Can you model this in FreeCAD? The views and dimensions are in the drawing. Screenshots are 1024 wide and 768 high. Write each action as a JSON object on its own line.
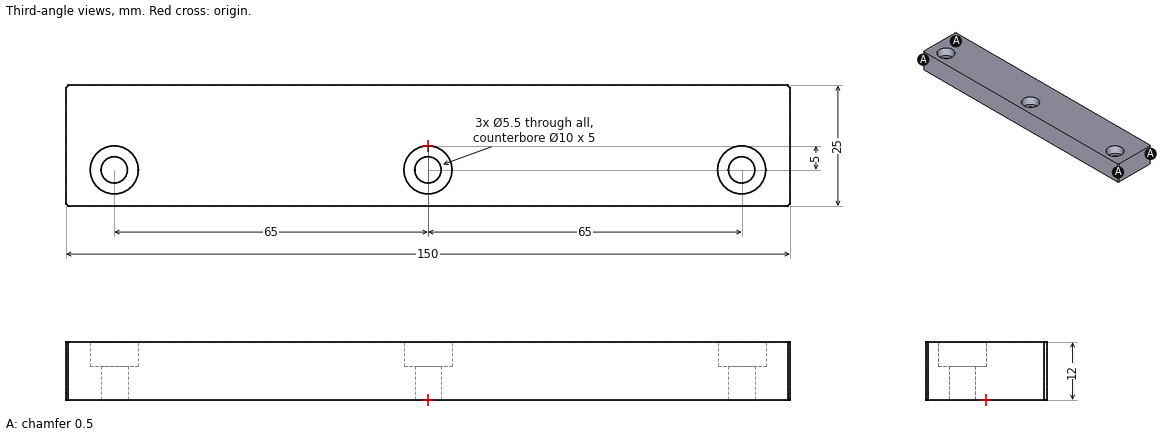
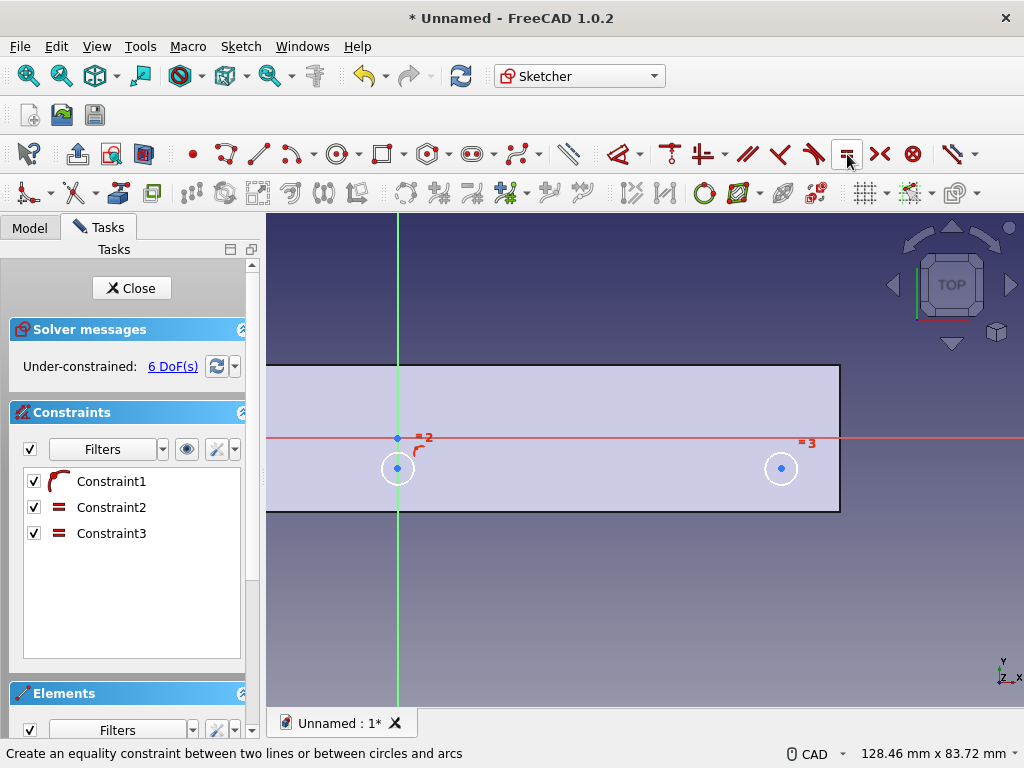
{"action": "left_click", "coordinate": [398, 469]}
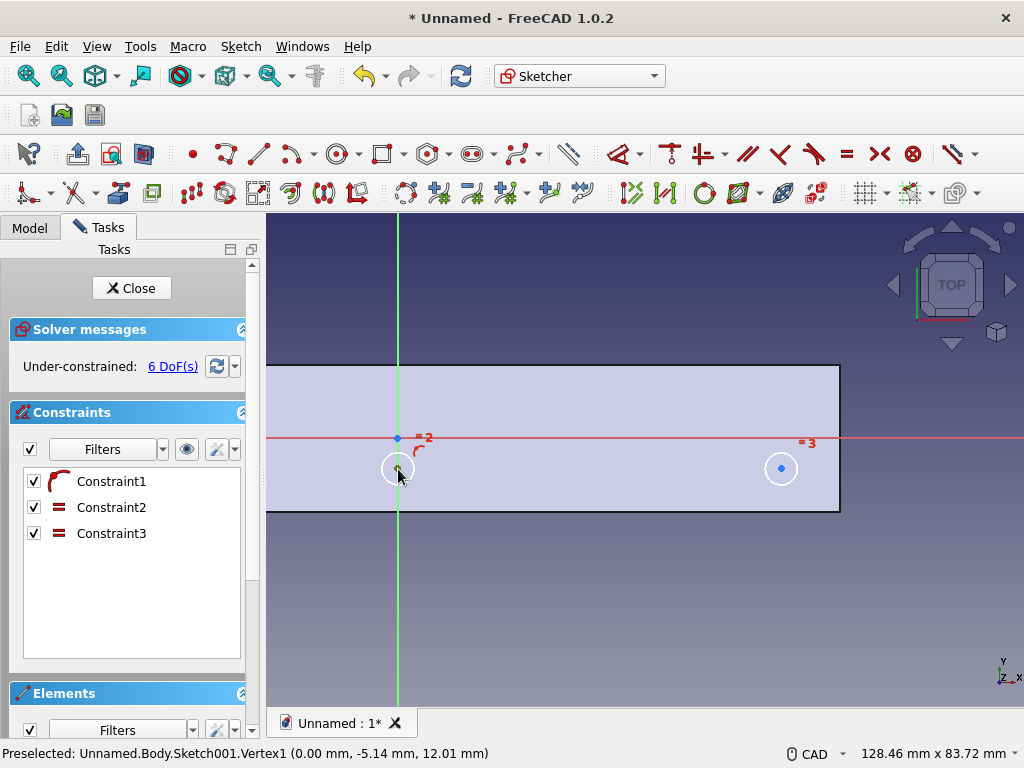
{"action": "scroll", "coordinate": [794, 458], "scroll_direction": "down", "scroll_amount": 3}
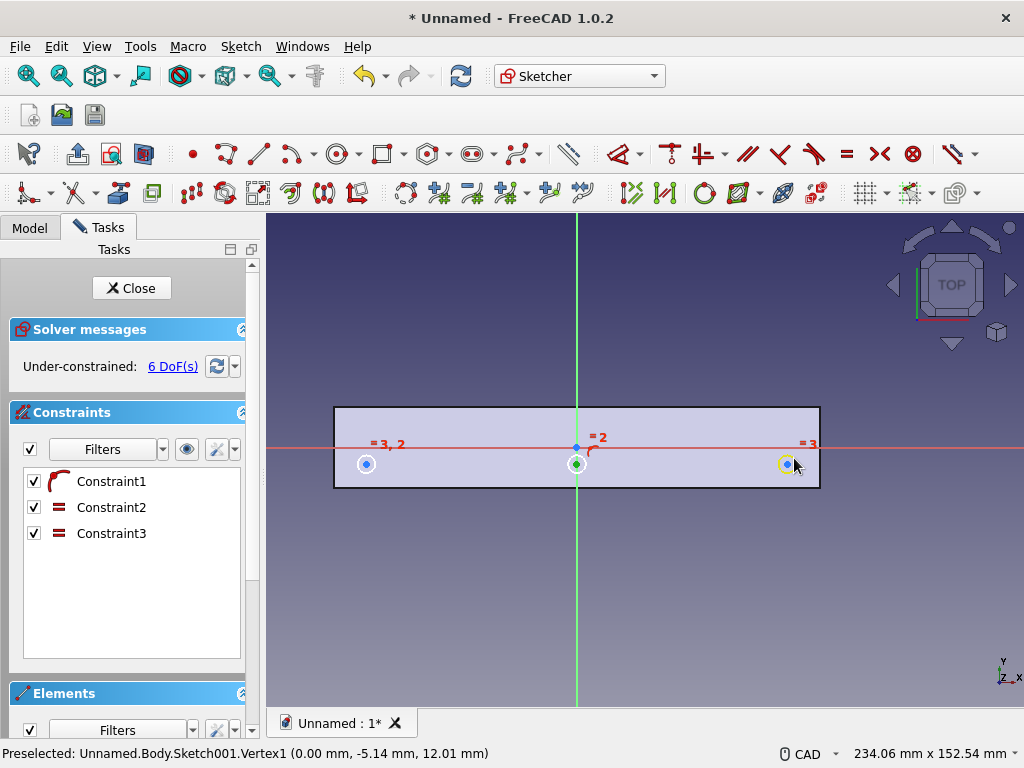
{"action": "left_click", "coordinate": [366, 464]}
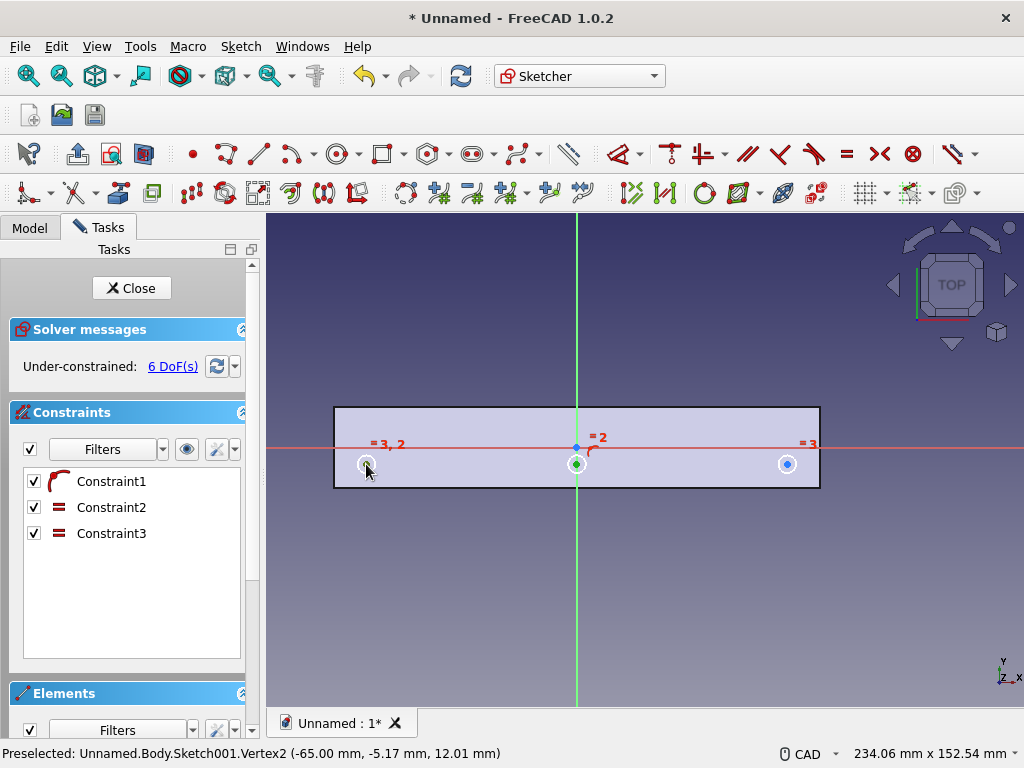
{"action": "left_click", "coordinate": [724, 154]}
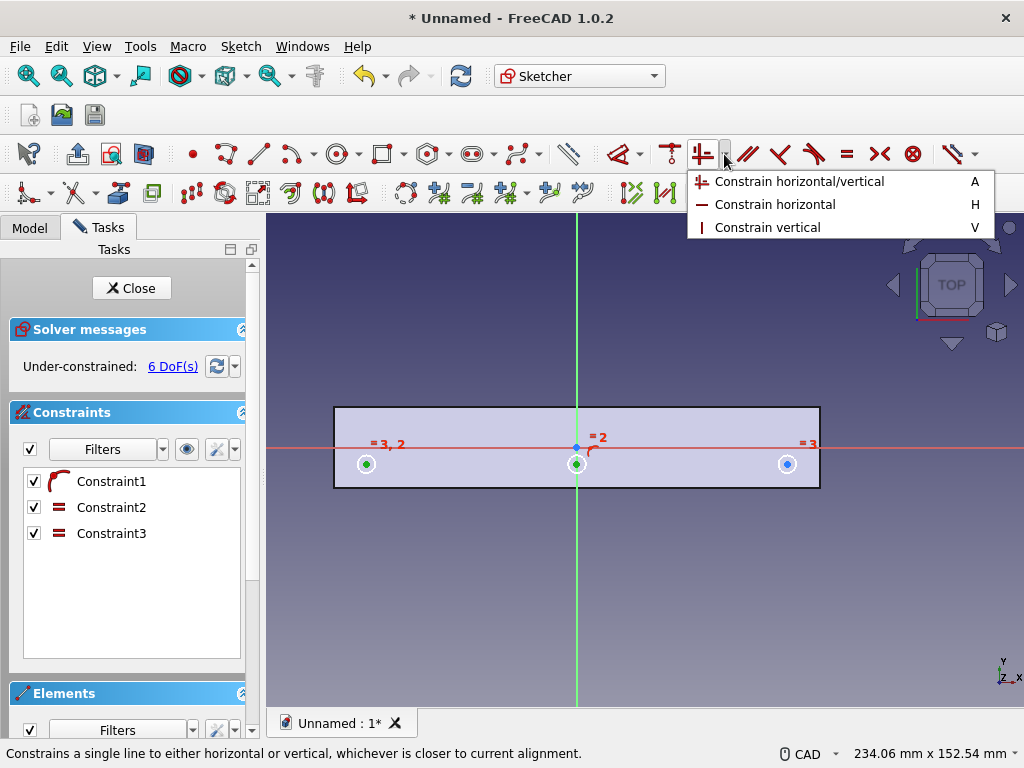
{"action": "left_click", "coordinate": [841, 204]}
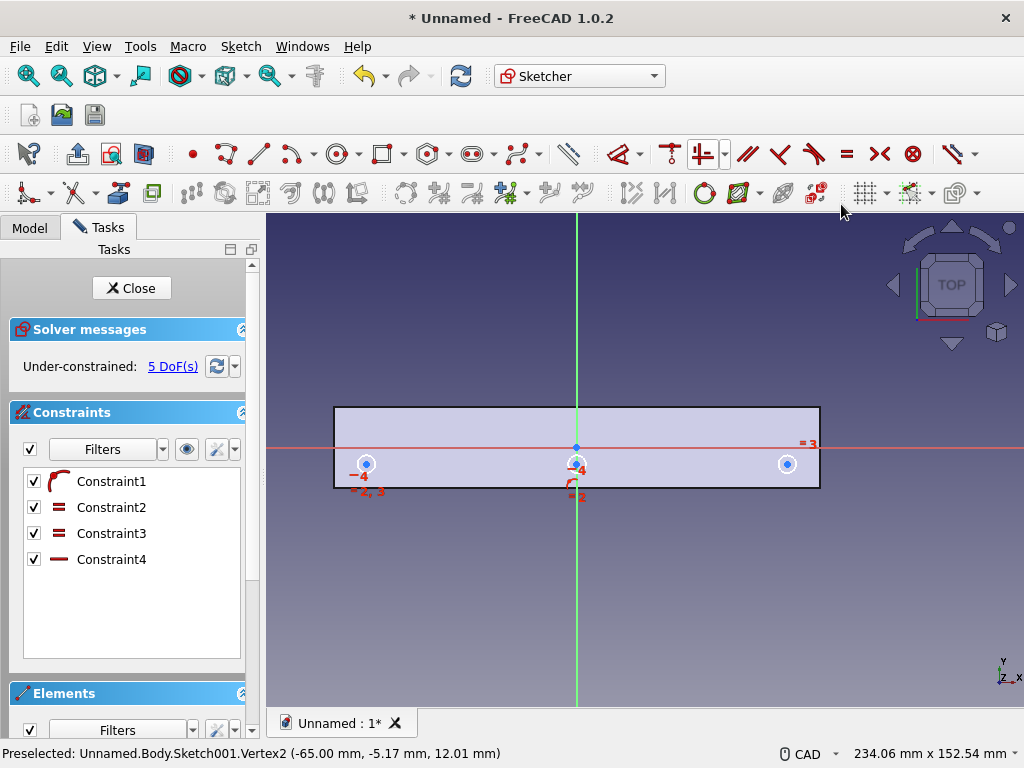
{"action": "left_click", "coordinate": [577, 464]}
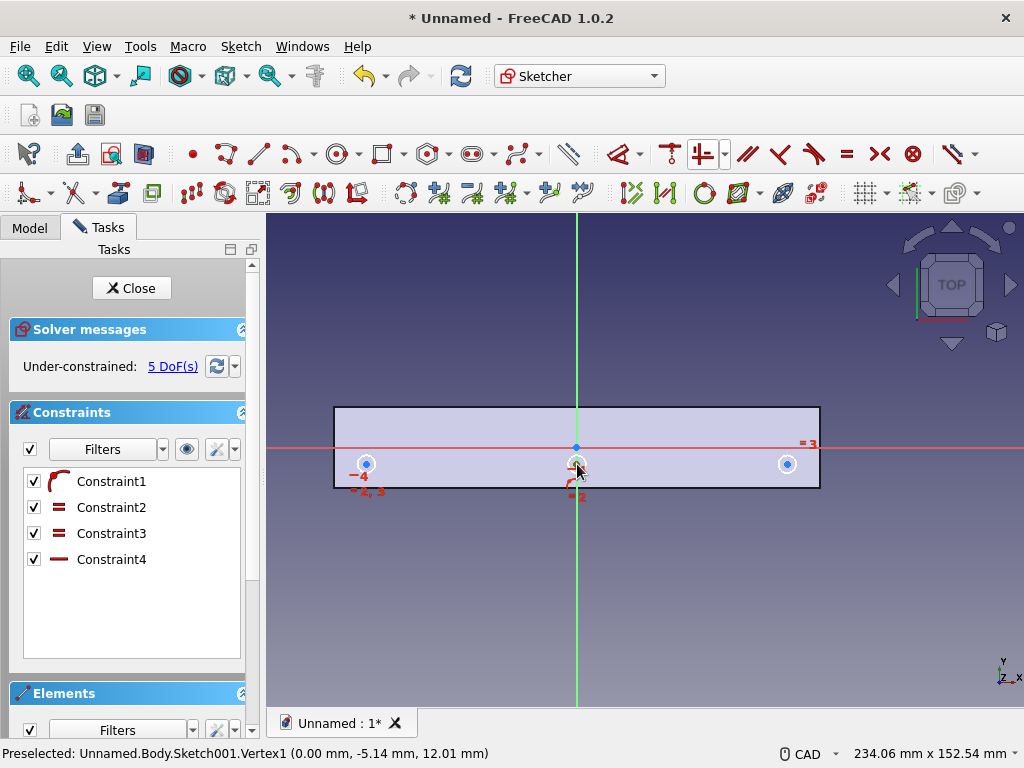
{"action": "left_click", "coordinate": [787, 464]}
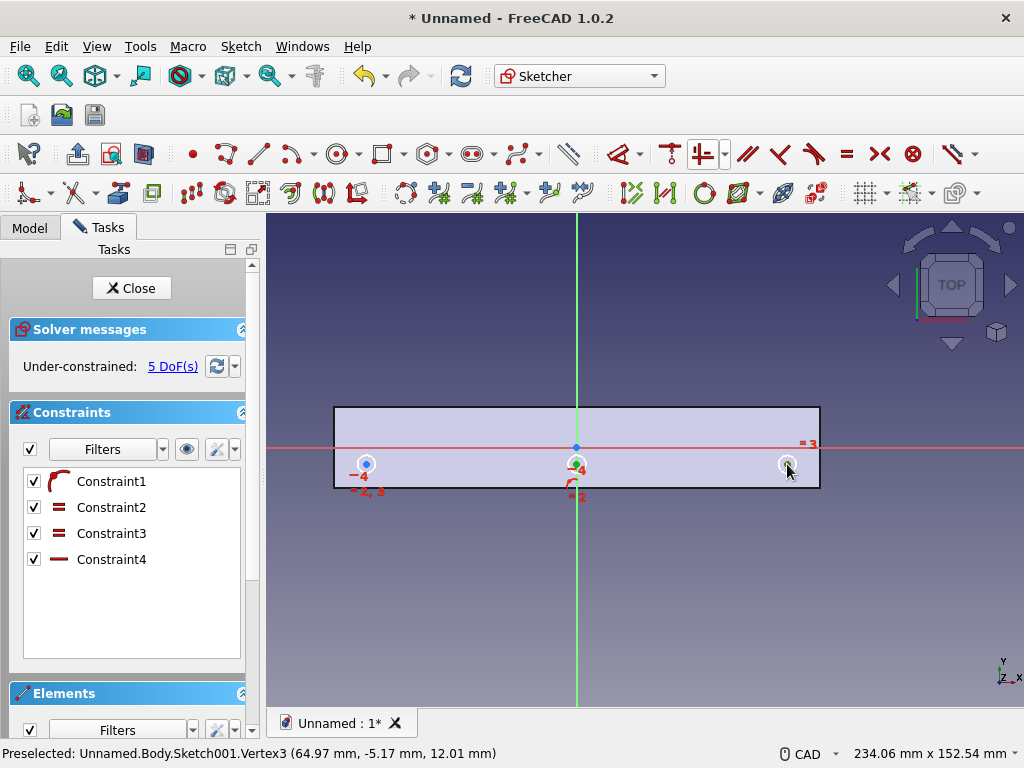
{"action": "left_click", "coordinate": [724, 154]}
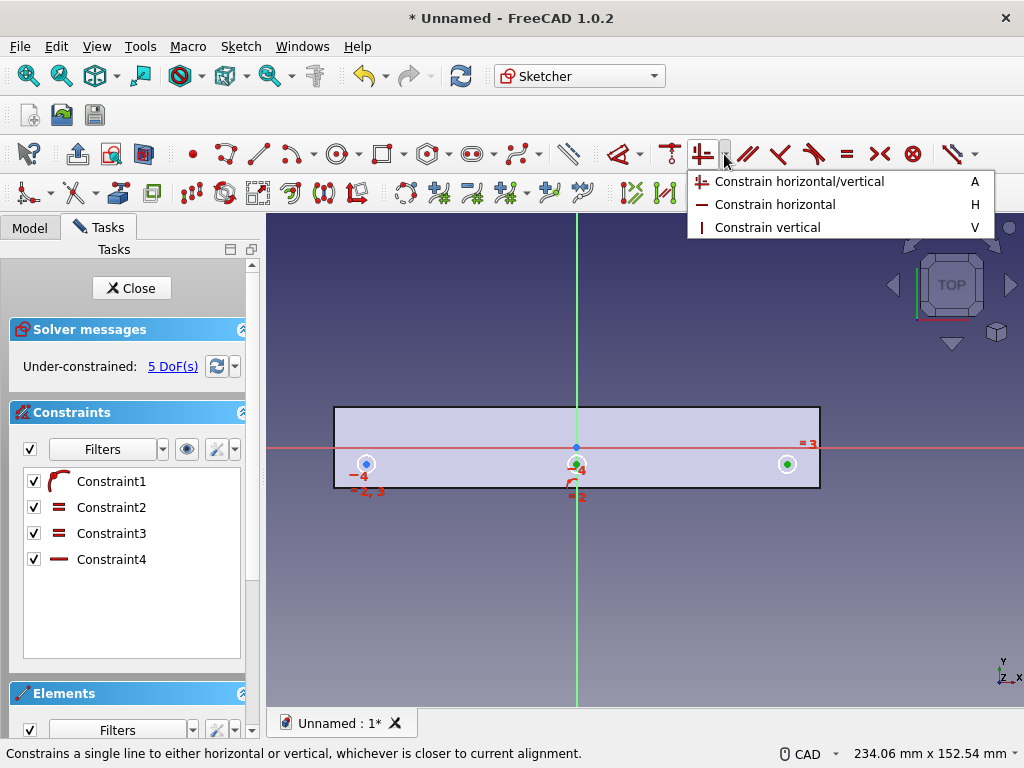
{"action": "left_click", "coordinate": [841, 204]}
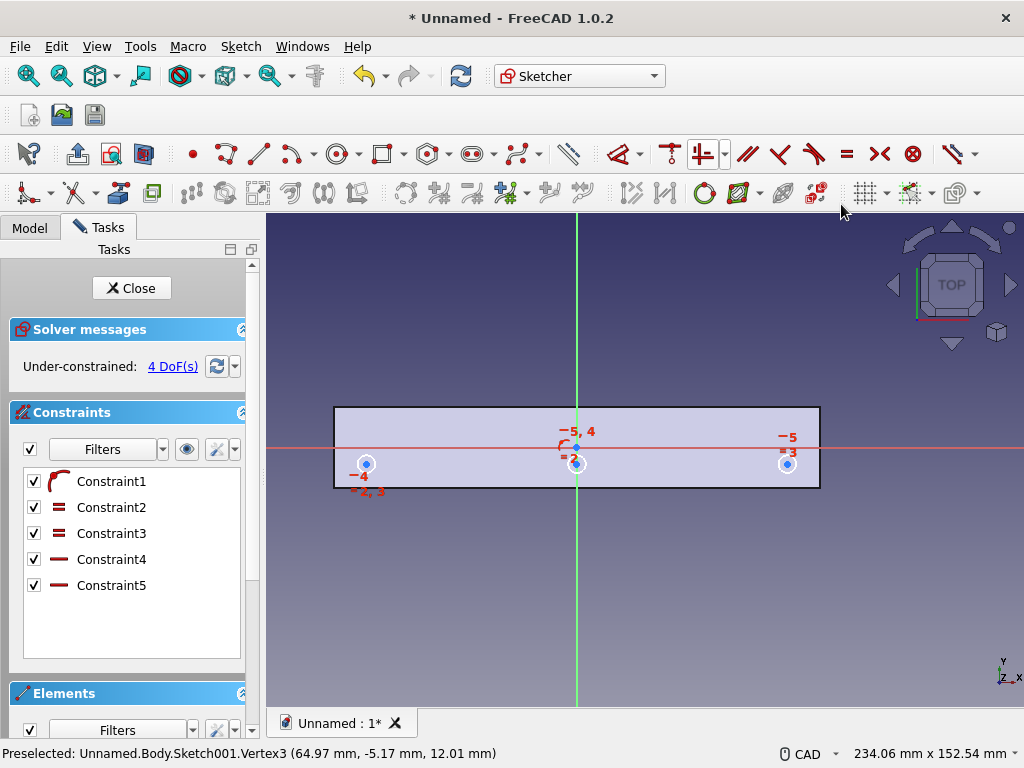
{"action": "left_click", "coordinate": [618, 154]}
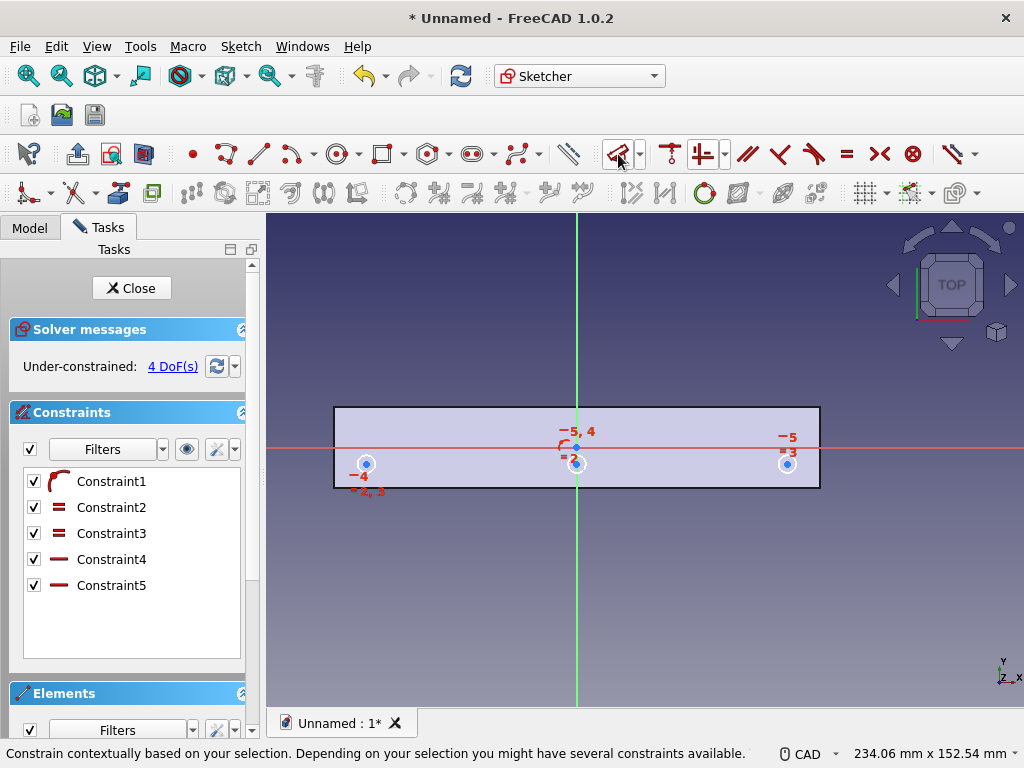
{"action": "scroll", "coordinate": [577, 473], "scroll_direction": "up", "scroll_amount": 5}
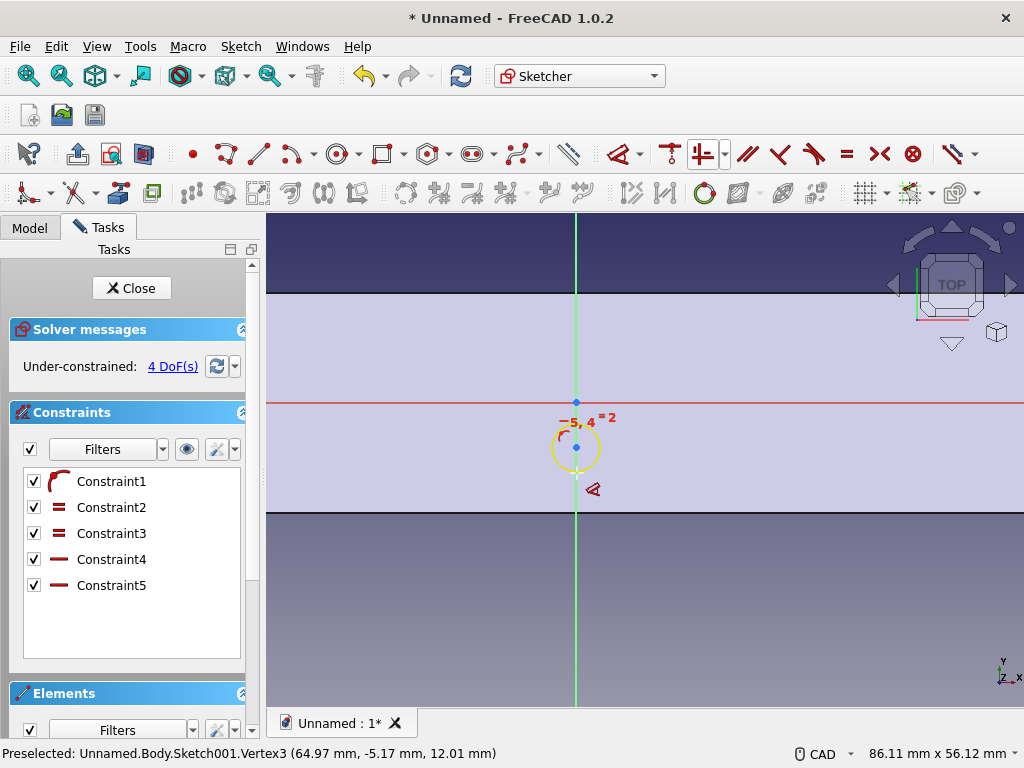
{"action": "left_click", "coordinate": [575, 472]}
{"action": "left_click", "coordinate": [547, 496]}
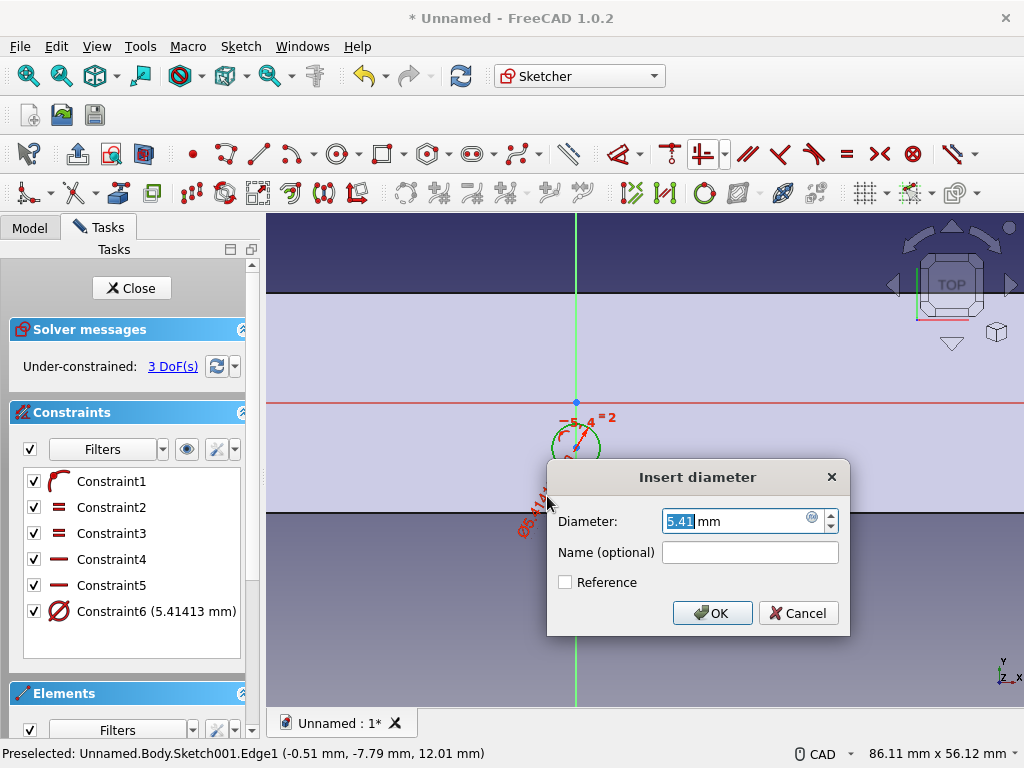
{"action": "type", "text": "5.5"}
{"action": "key", "text": "Return"}